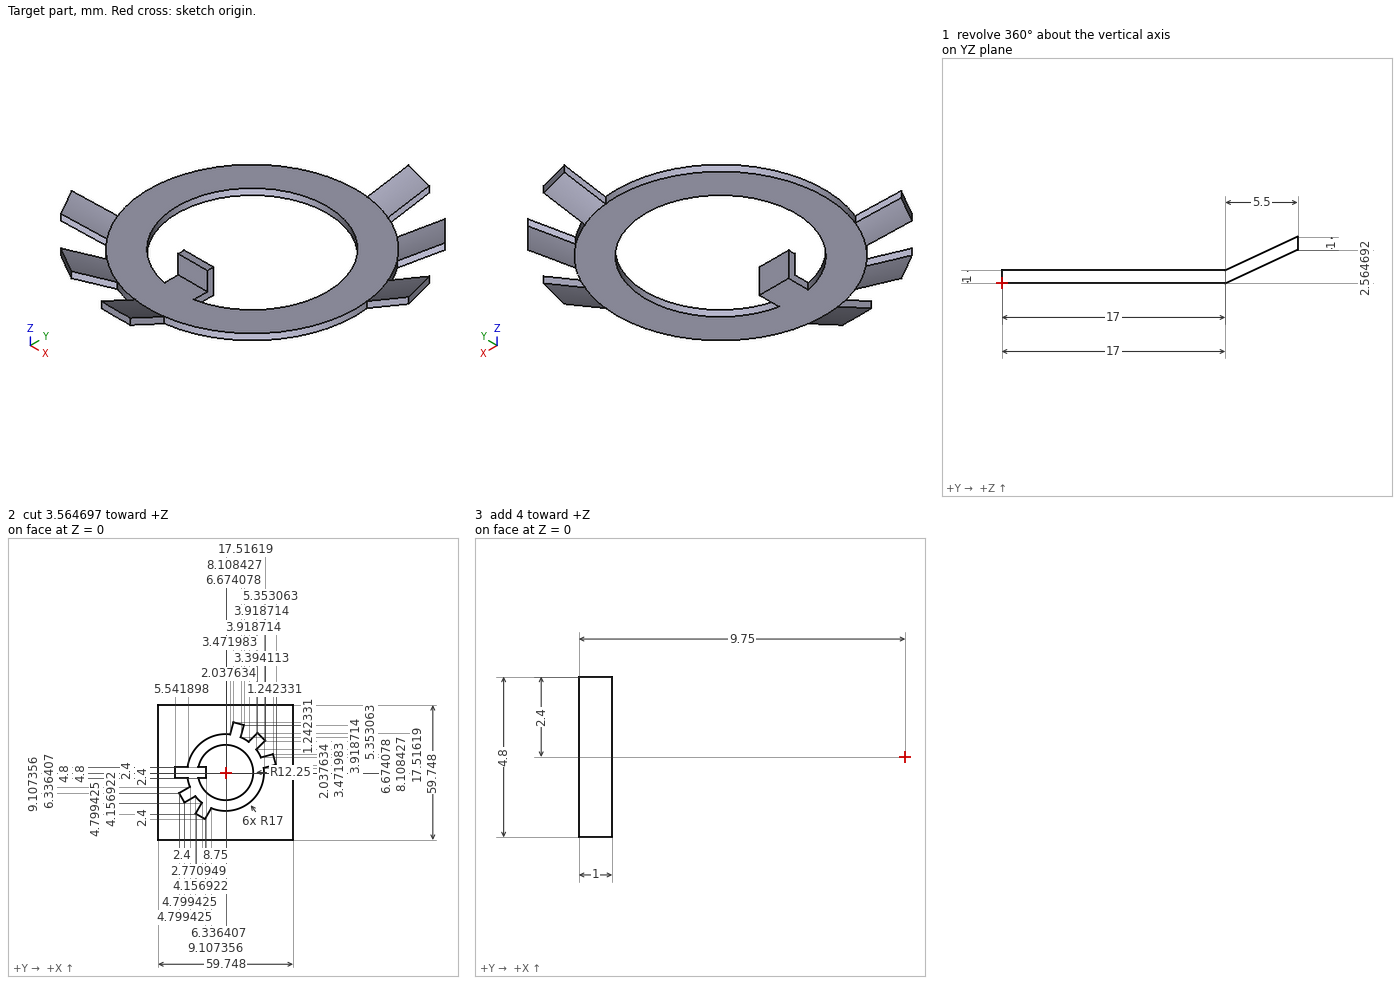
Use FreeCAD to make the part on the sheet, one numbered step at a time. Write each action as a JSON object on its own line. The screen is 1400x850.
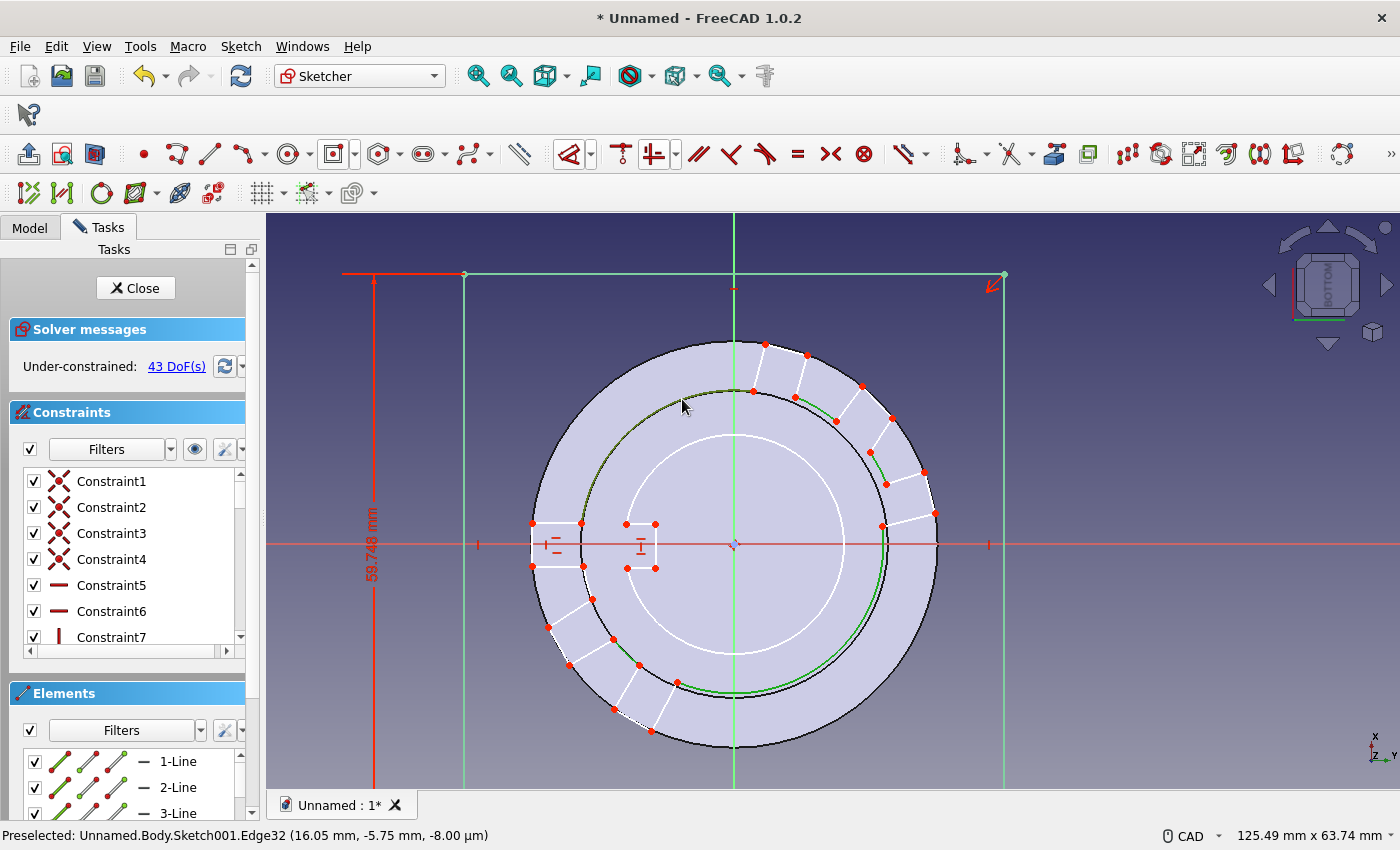
{"action": "scroll", "coordinate": [586, 577], "scroll_direction": "up", "scroll_amount": 2}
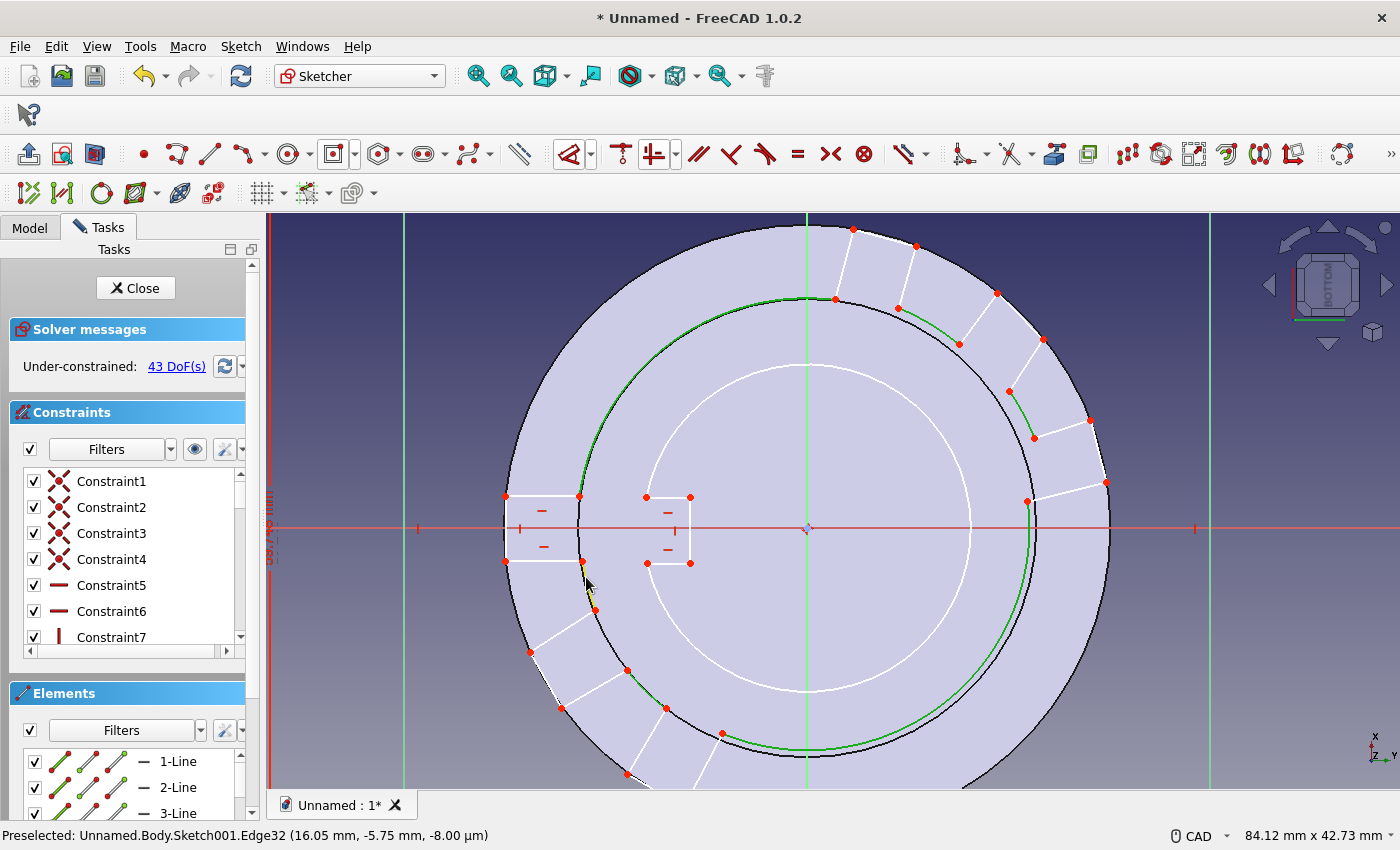
{"action": "left_click", "coordinate": [585, 576]}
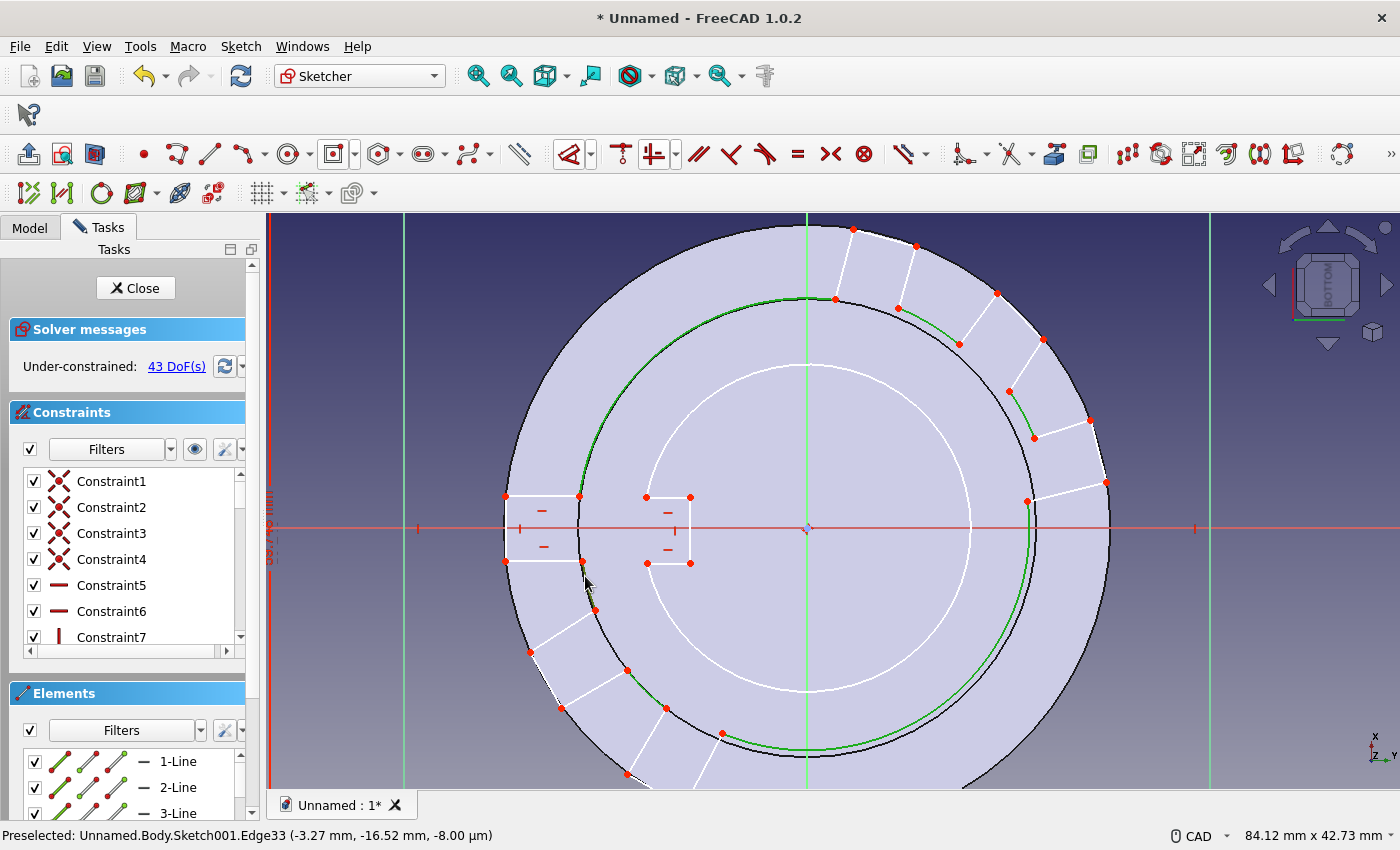
{"action": "left_click", "coordinate": [798, 154]}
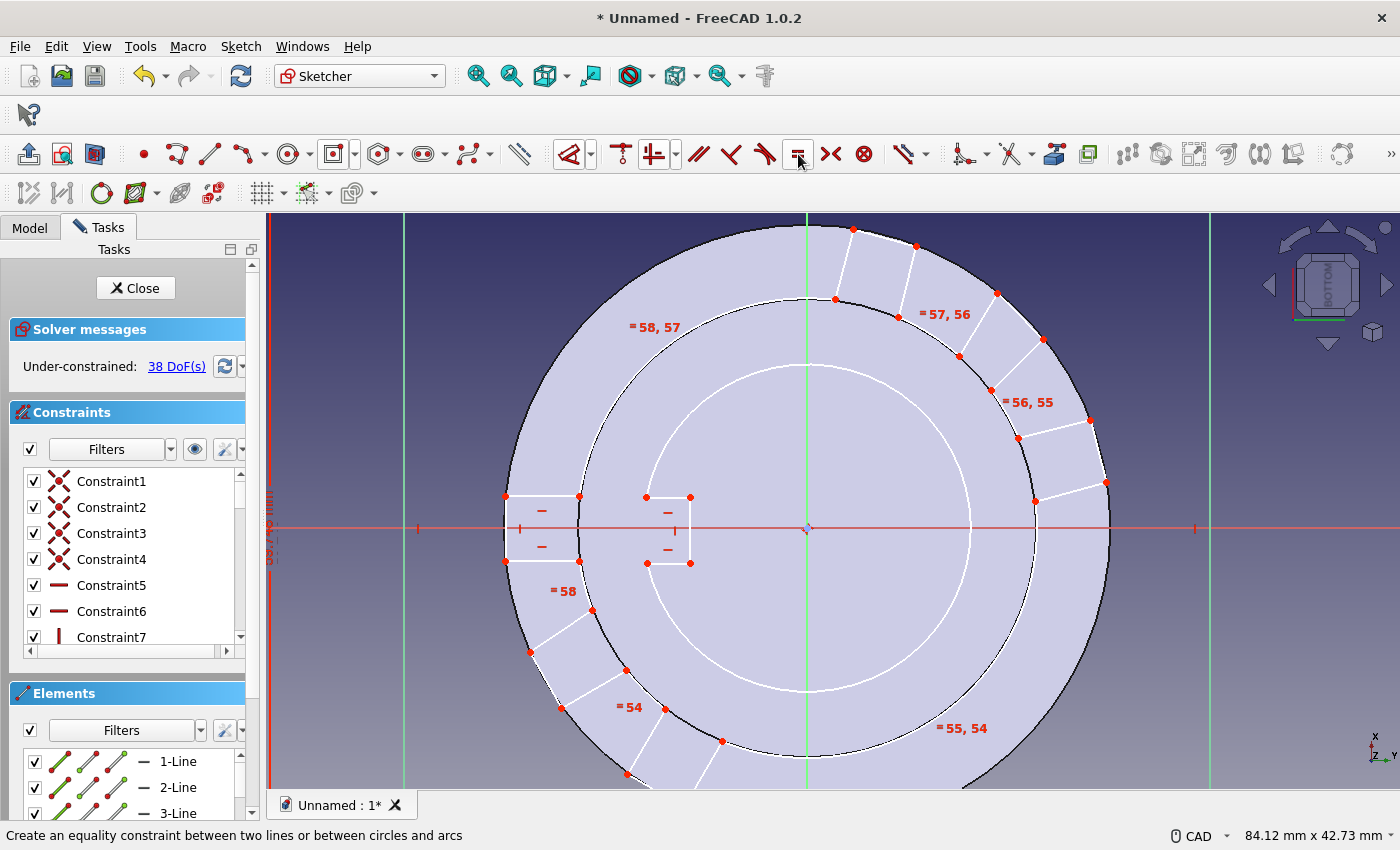
{"action": "left_click", "coordinate": [873, 678]}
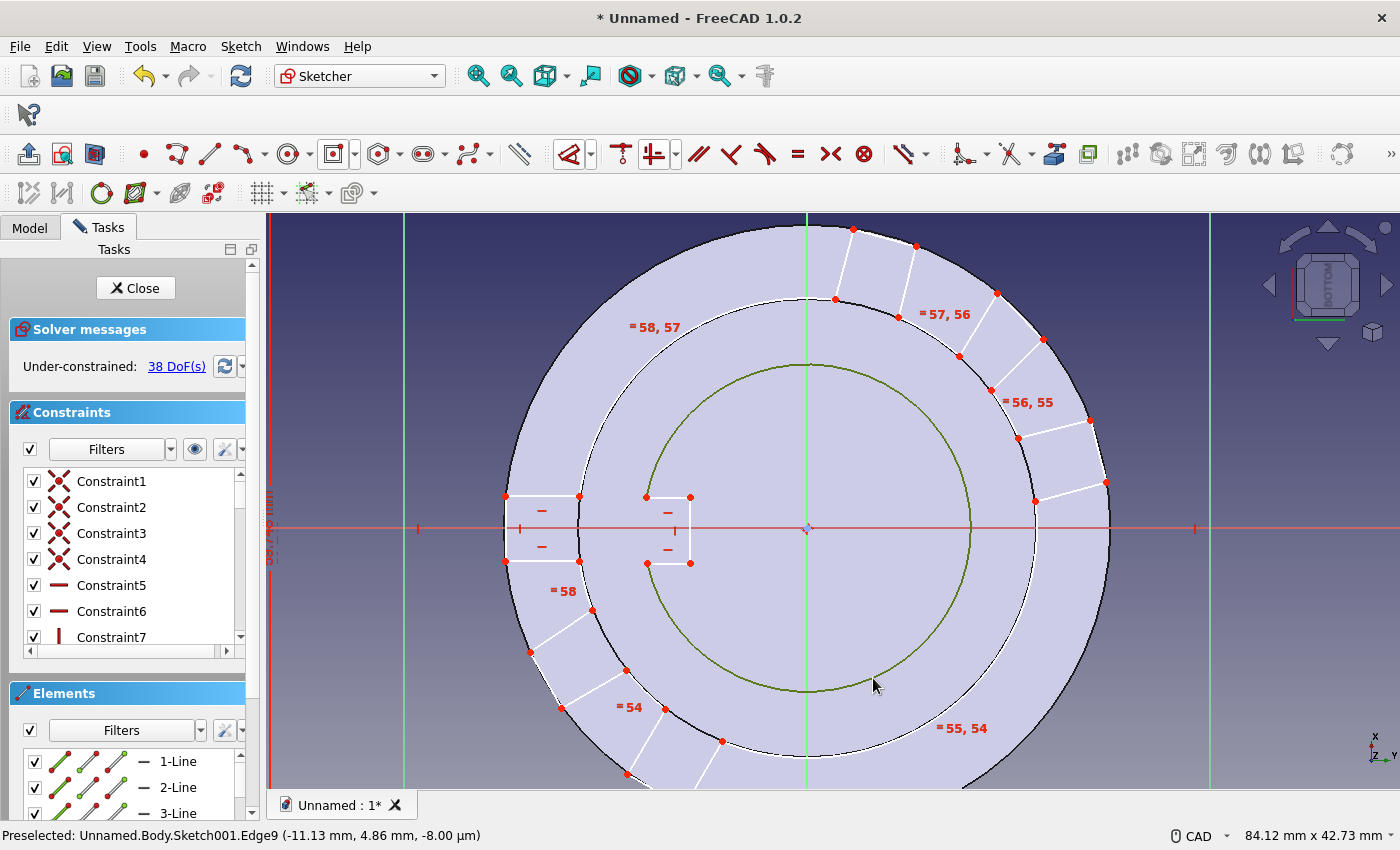
{"action": "key", "text": "k r"}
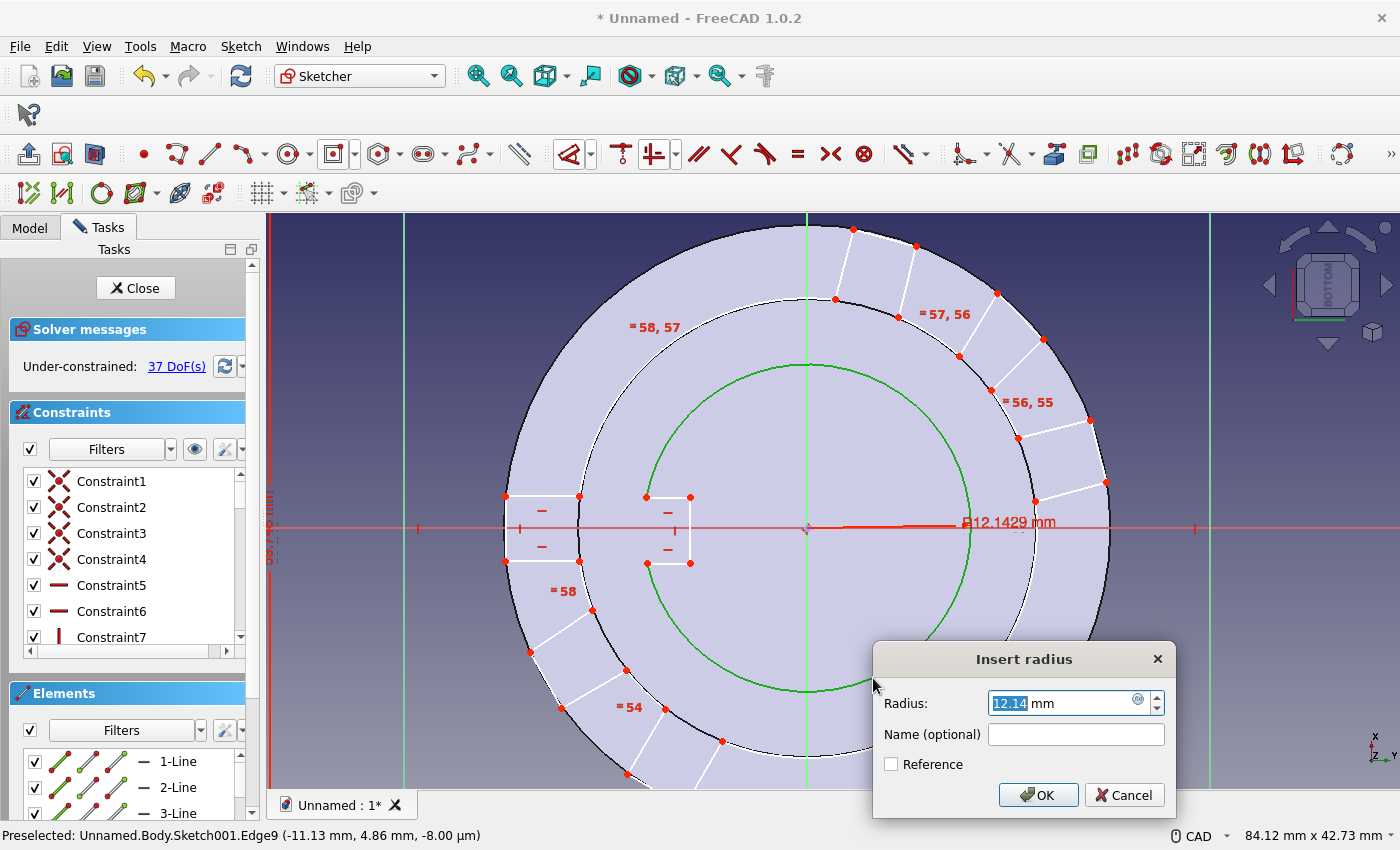
{"action": "type", "text": "12.25"}
{"action": "key", "text": "Return"}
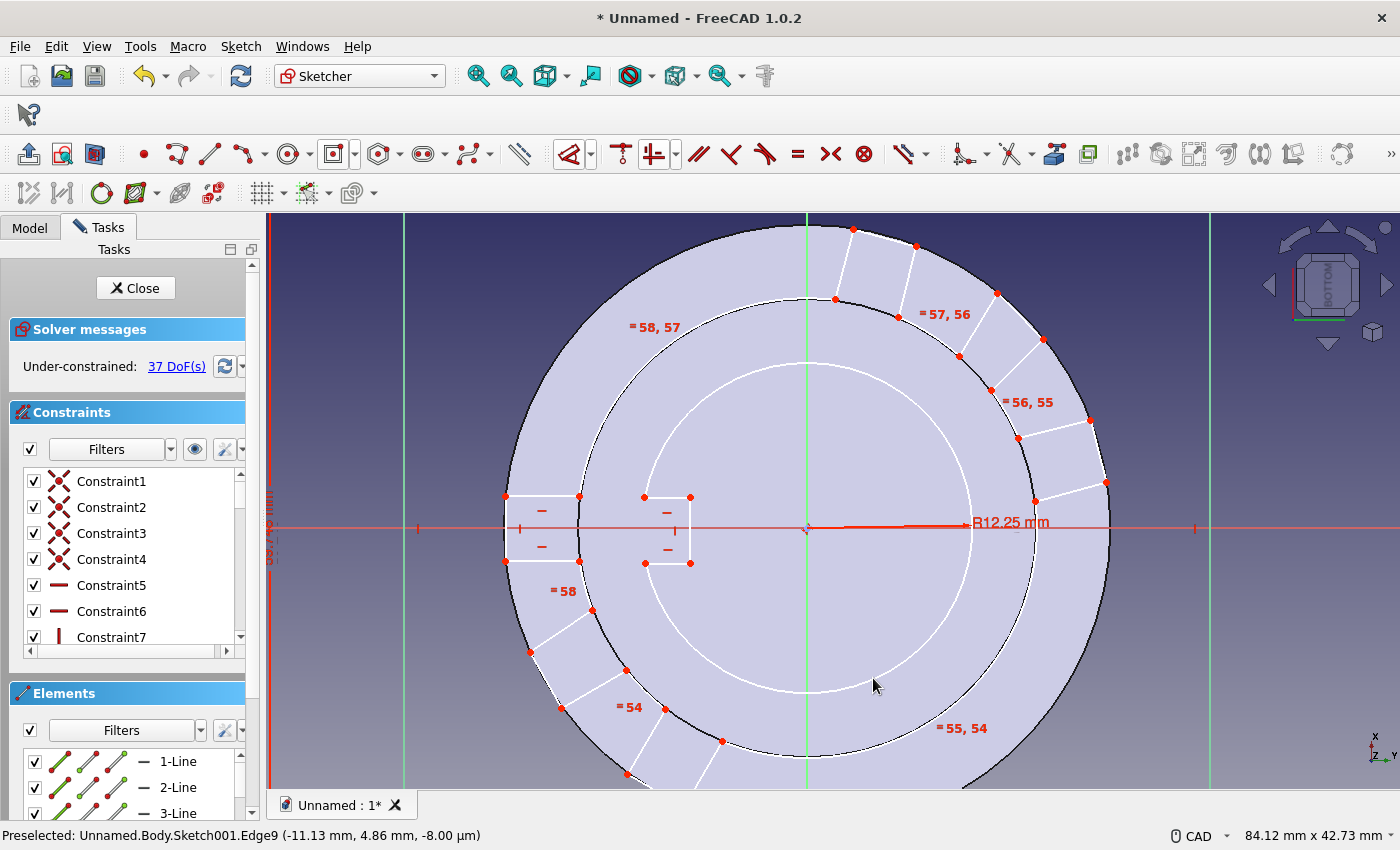
{"action": "left_click", "coordinate": [637, 683]}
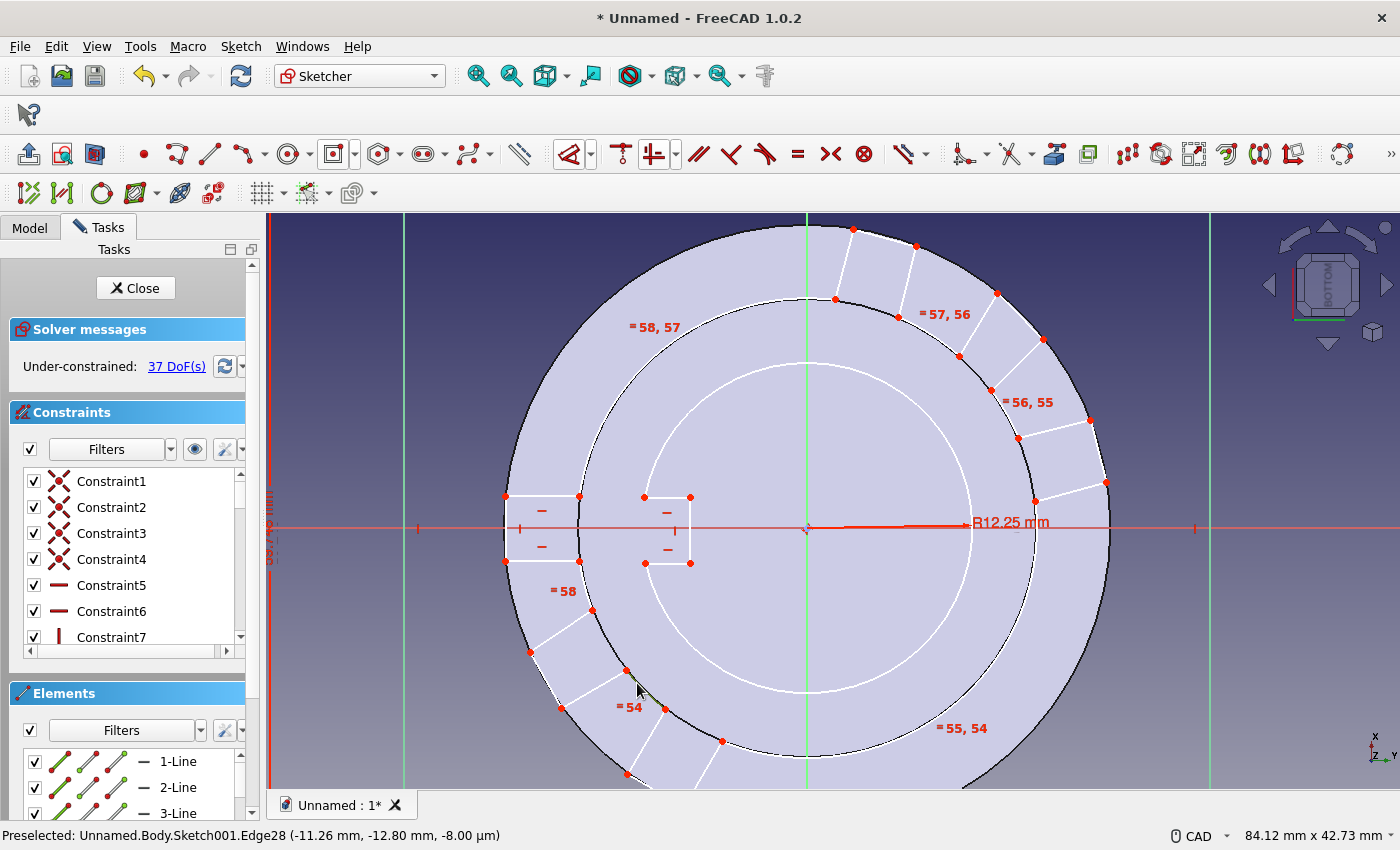
{"action": "key", "text": "k r"}